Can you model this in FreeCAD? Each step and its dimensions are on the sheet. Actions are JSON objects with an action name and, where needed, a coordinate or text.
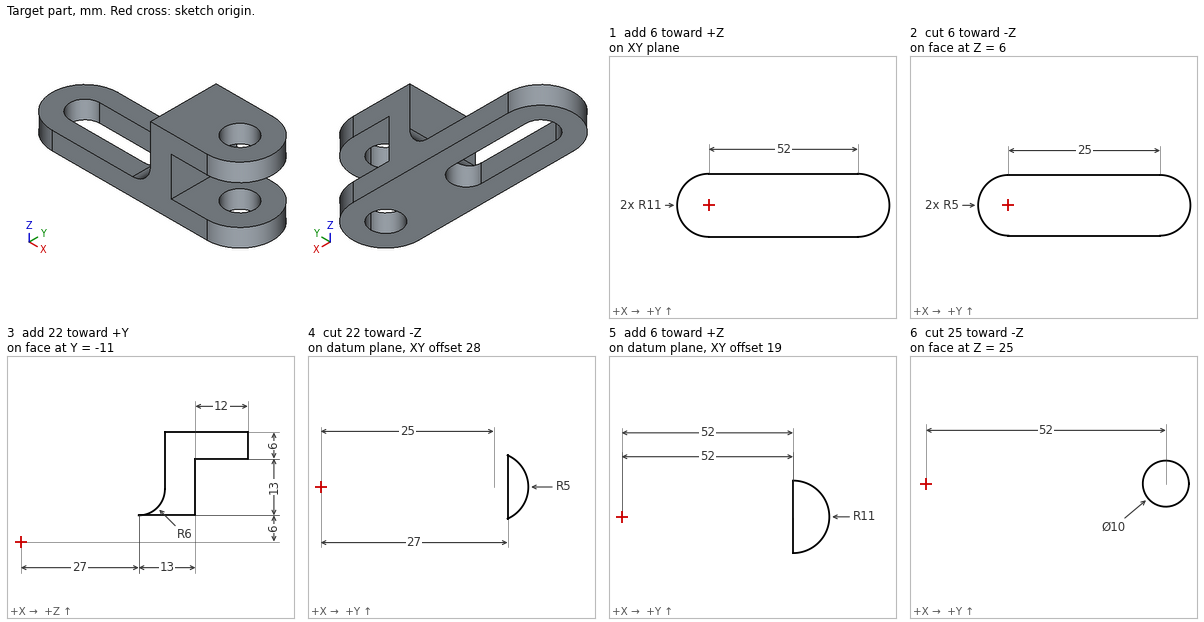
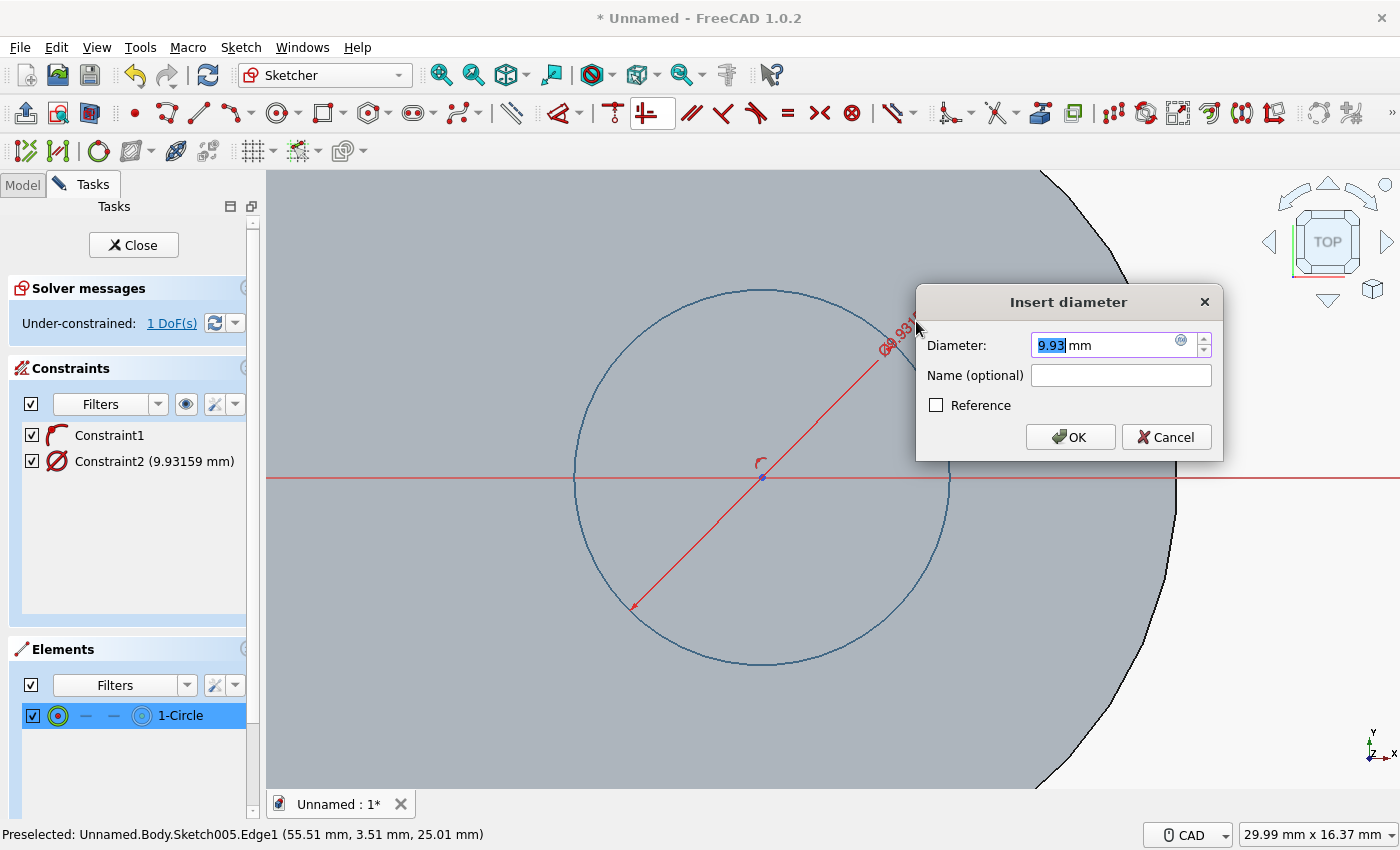
{"action": "type", "text": "10"}
{"action": "key", "text": "Return"}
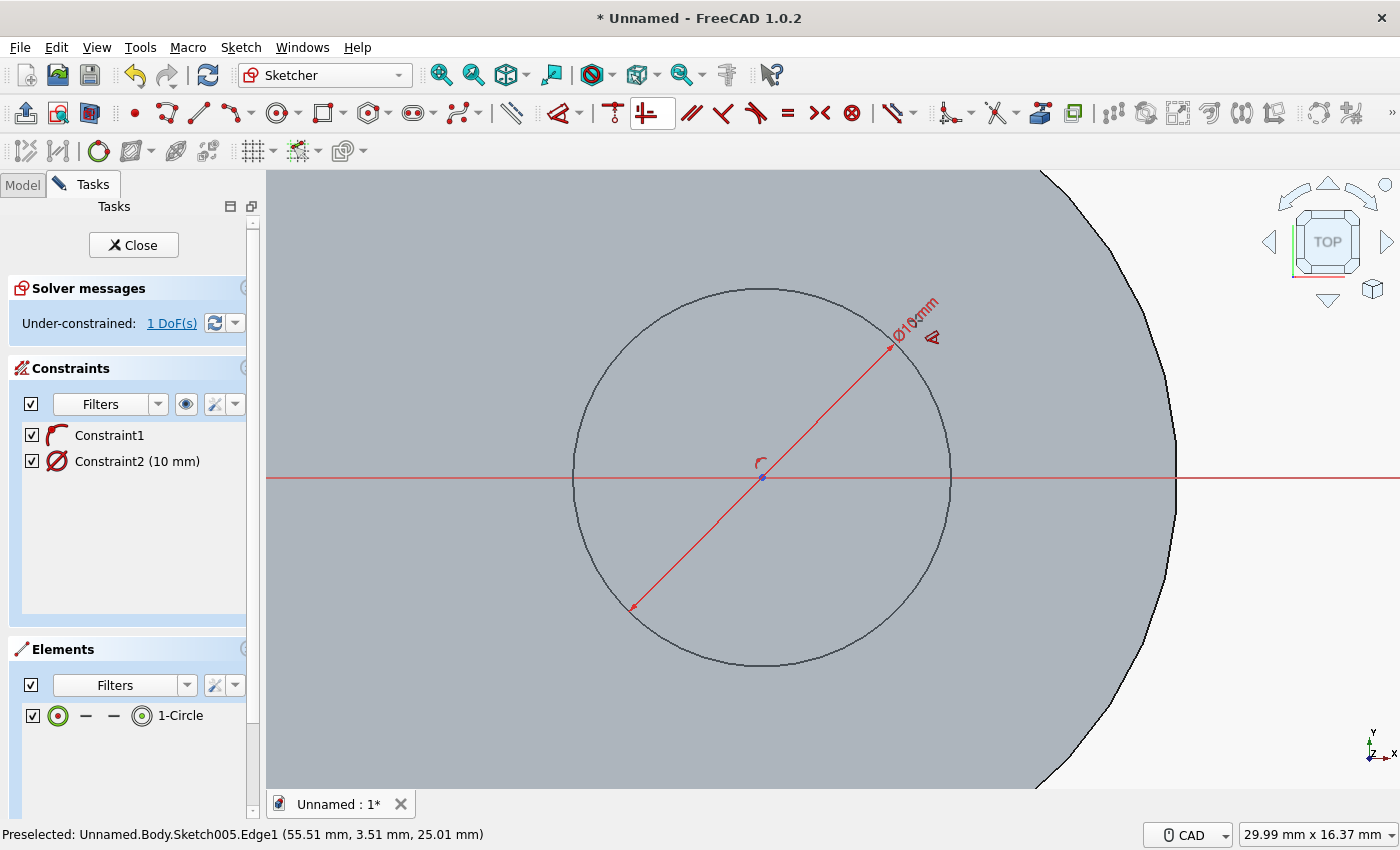
{"action": "left_click", "coordinate": [762, 478]}
{"action": "left_click", "coordinate": [528, 512]}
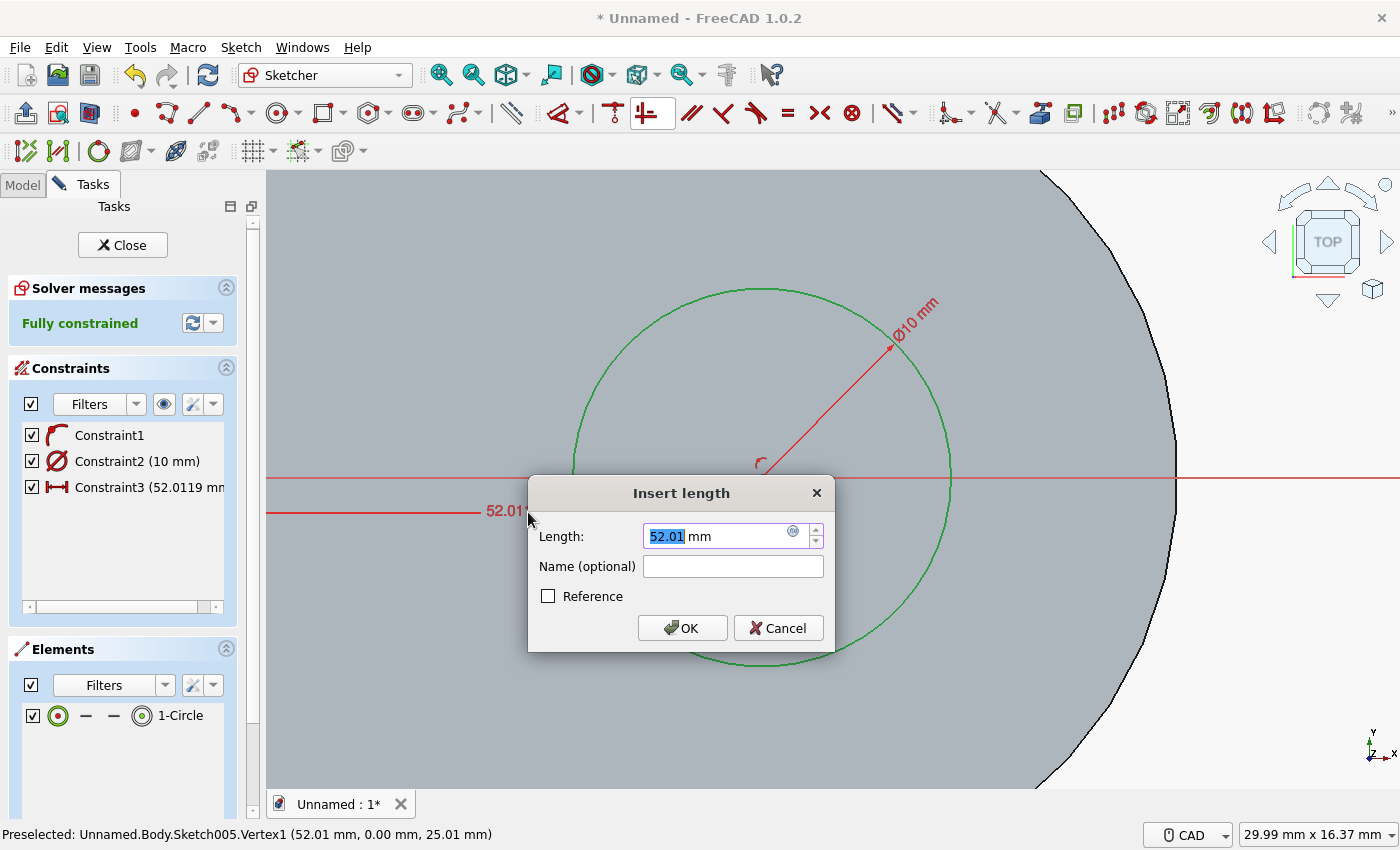
{"action": "type", "text": "52"}
{"action": "key", "text": "Return"}
{"action": "key", "text": "Escape"}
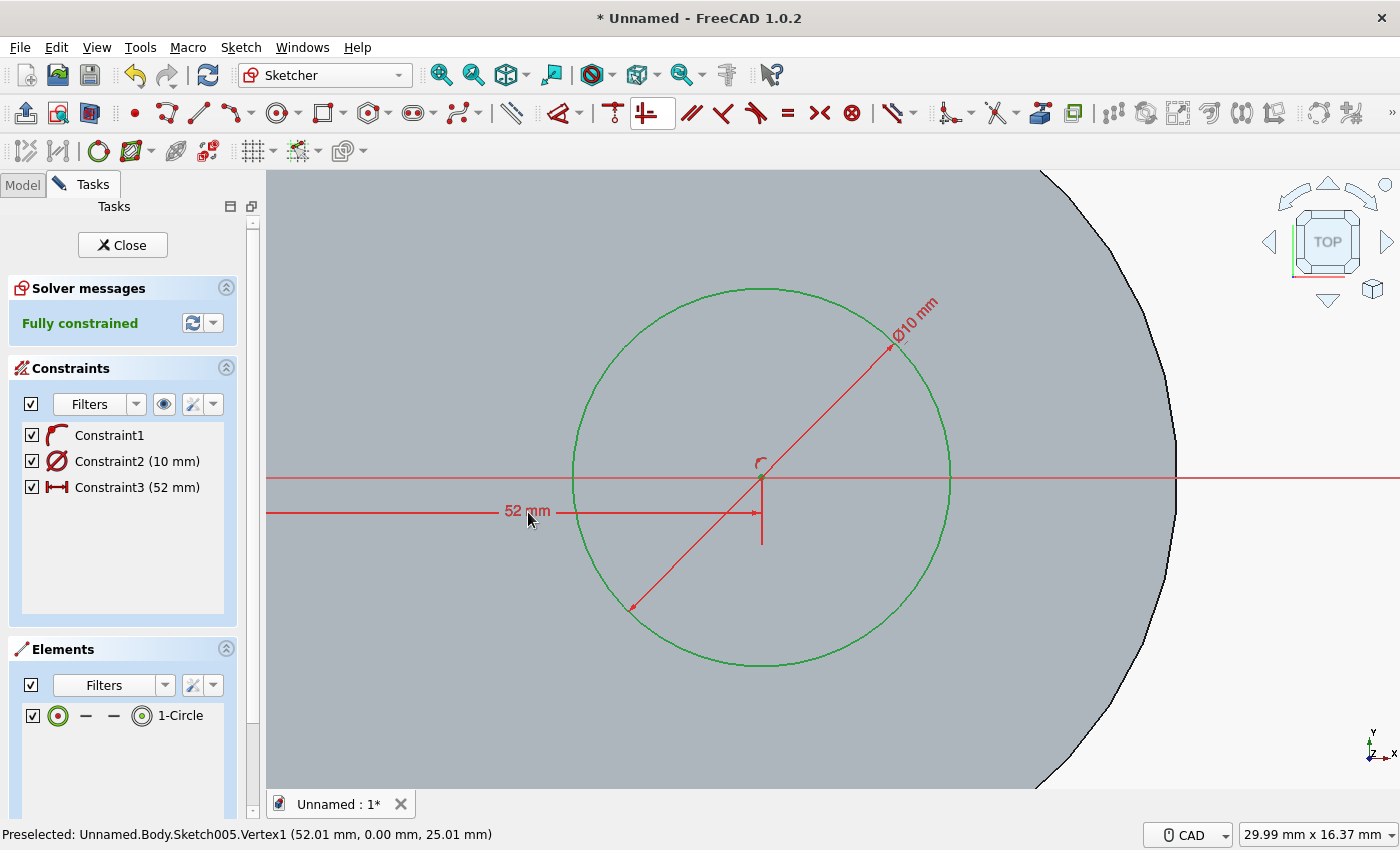
{"action": "left_click", "coordinate": [123, 245]}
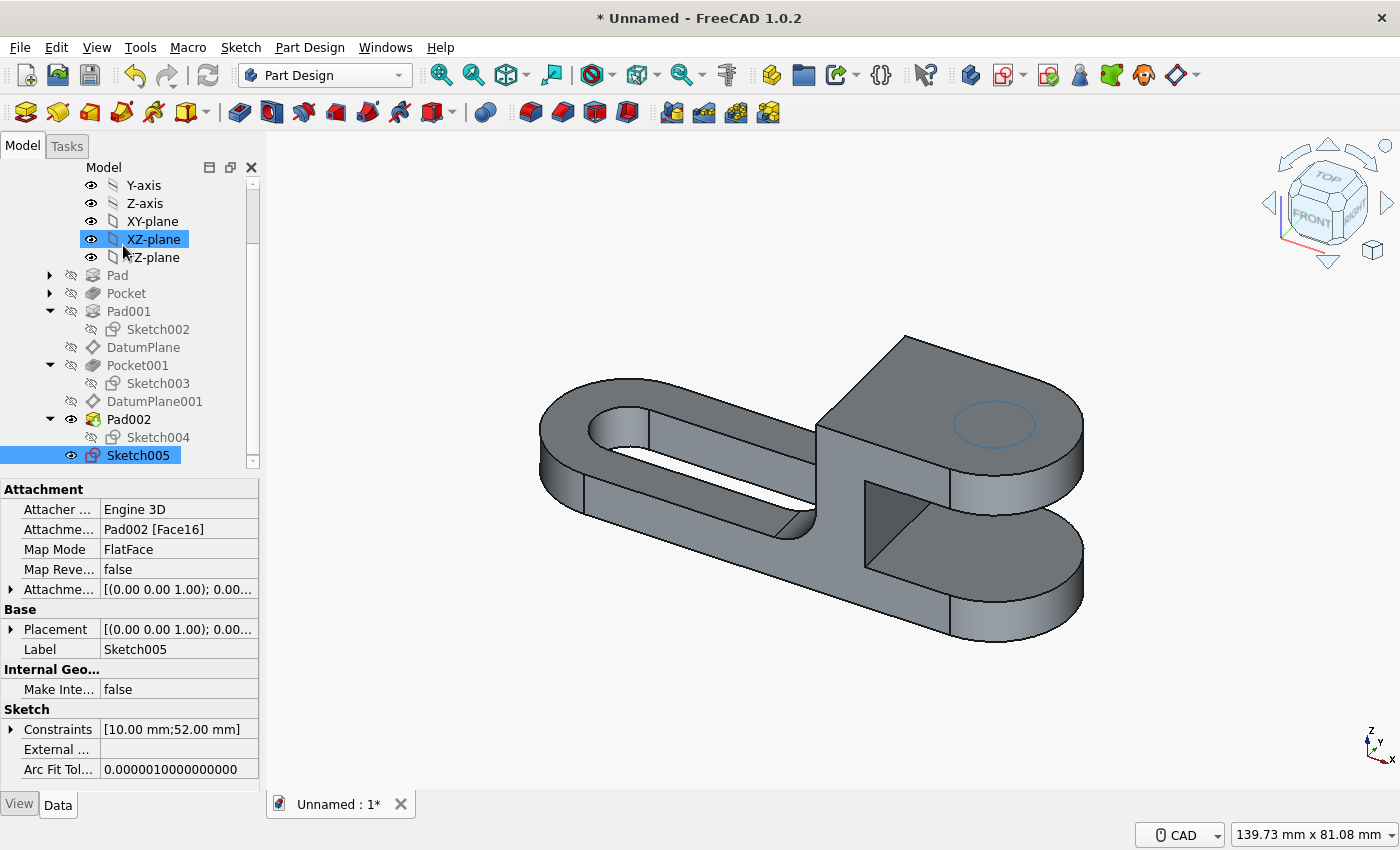
{"action": "left_click", "coordinate": [240, 112]}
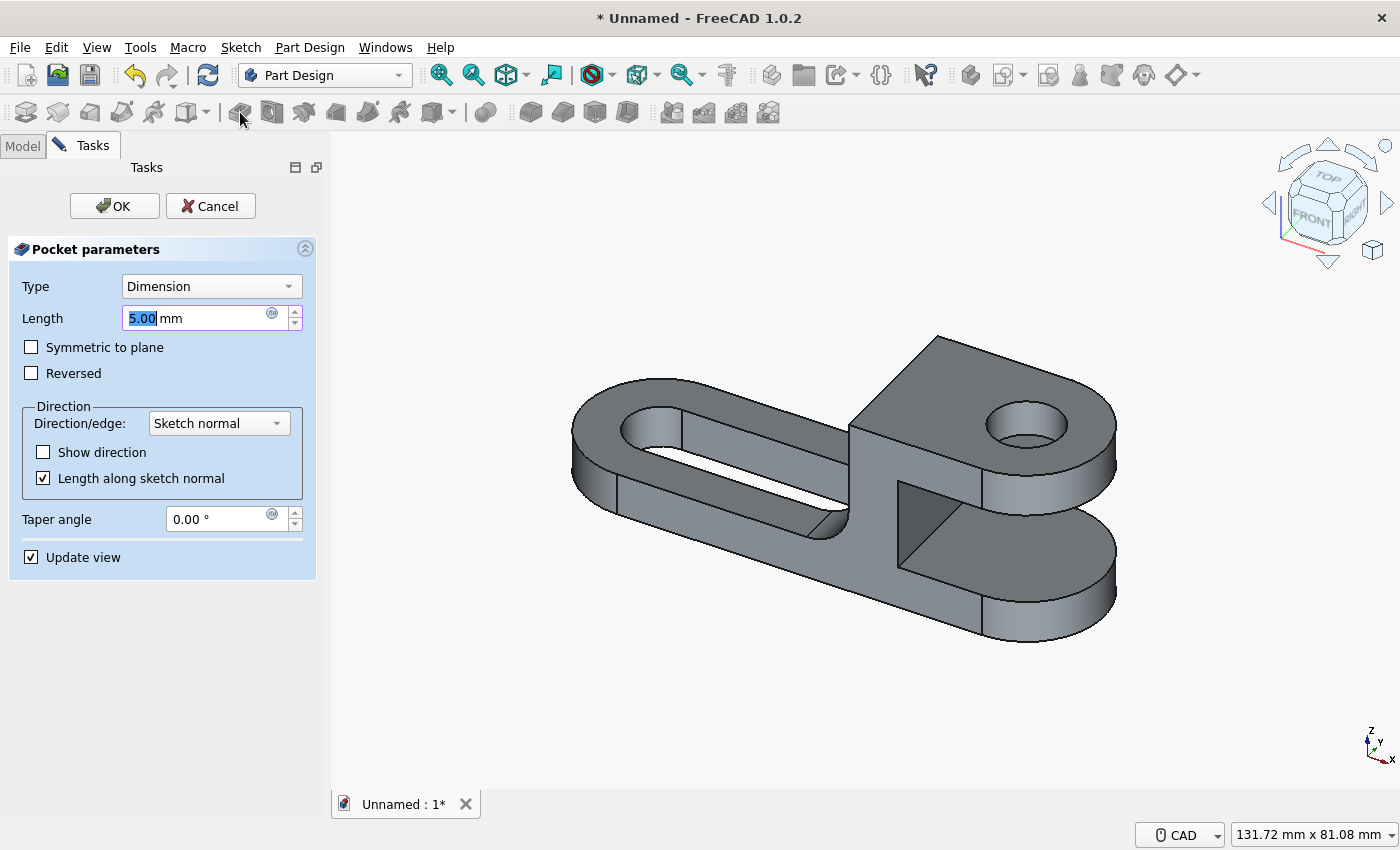
{"action": "type", "text": "25"}
{"action": "key", "text": "Tab"}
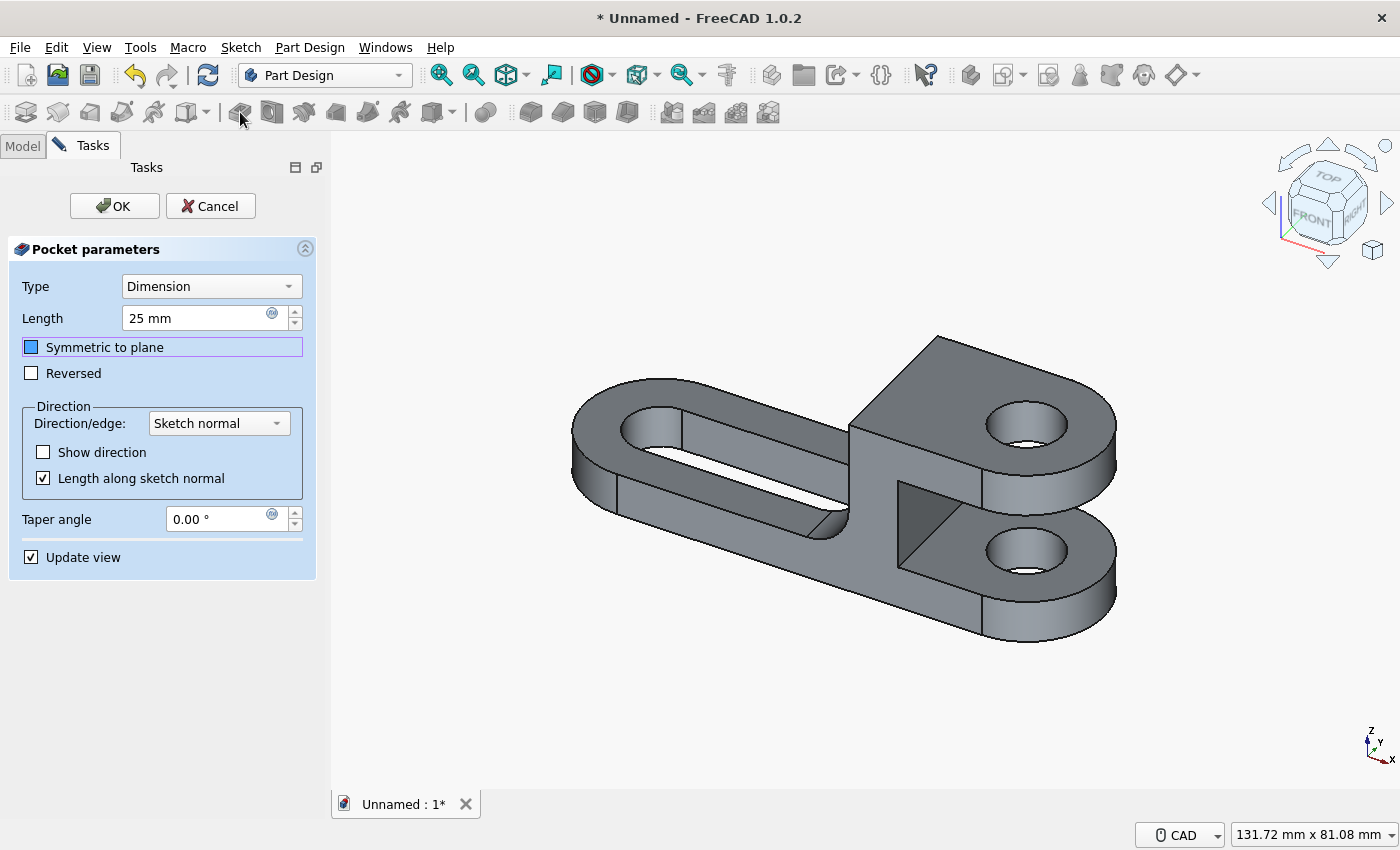
{"action": "left_click", "coordinate": [115, 206]}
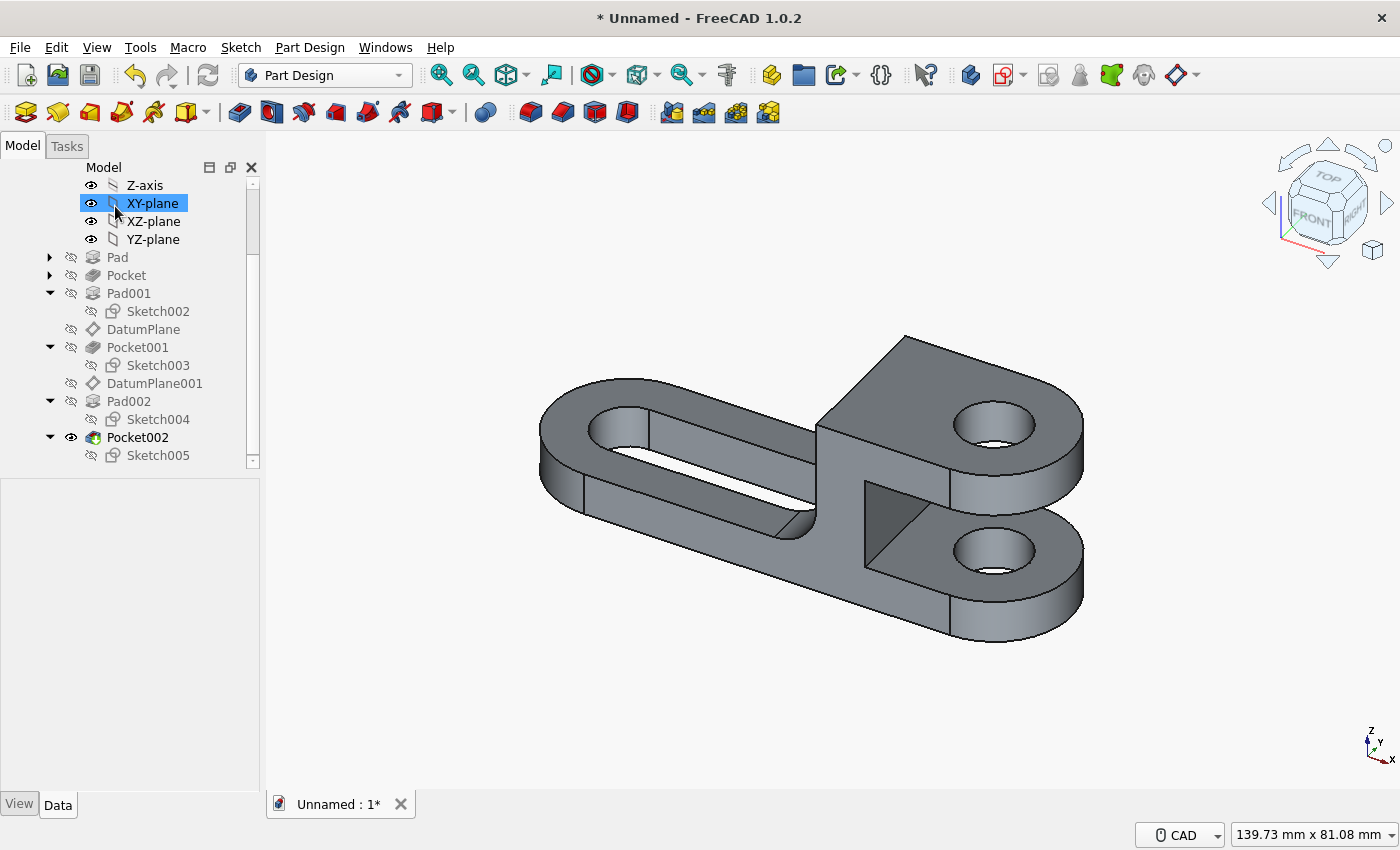
{"action": "key", "text": "0"}